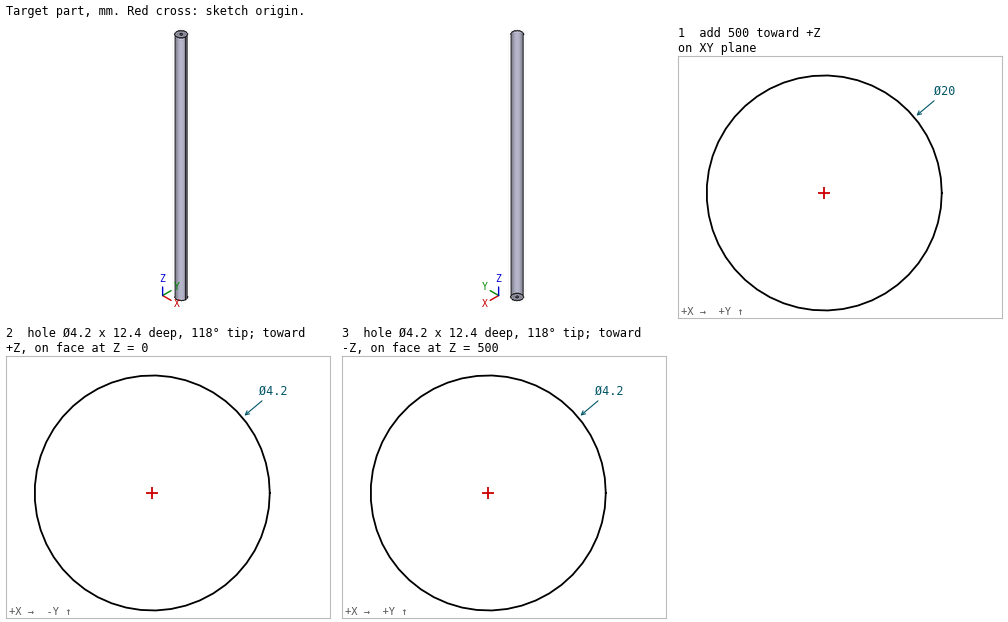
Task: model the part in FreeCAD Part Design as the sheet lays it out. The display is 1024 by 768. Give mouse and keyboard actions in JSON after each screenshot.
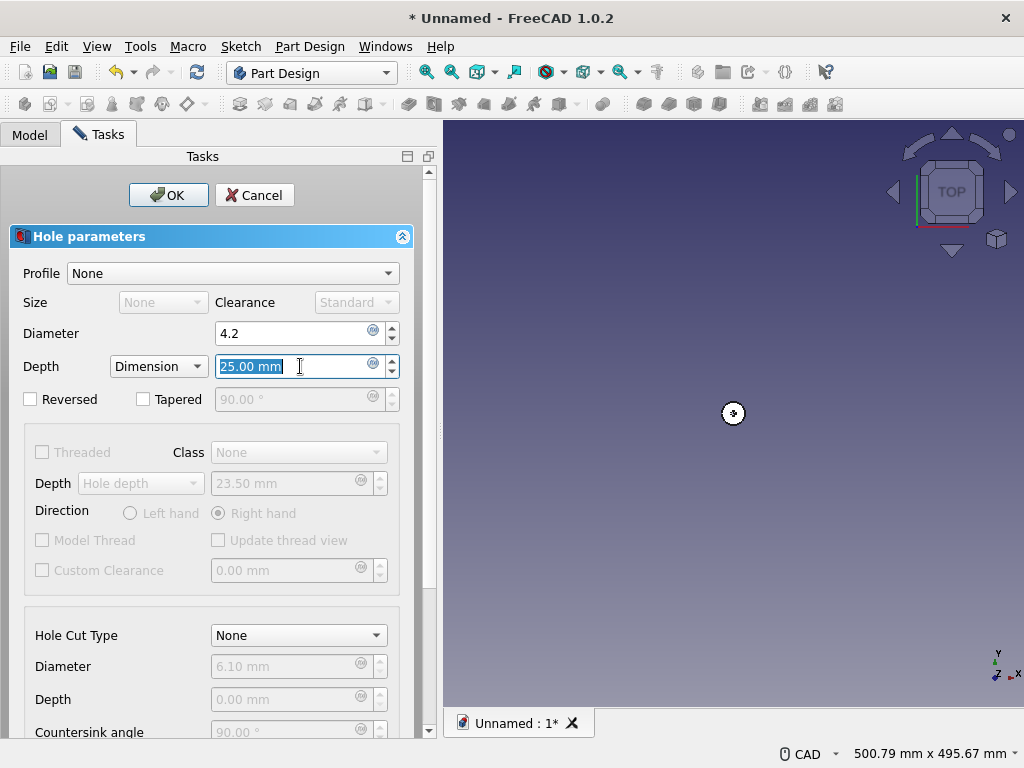
{"action": "type", "text": "12.4"}
{"action": "key", "text": "Tab"}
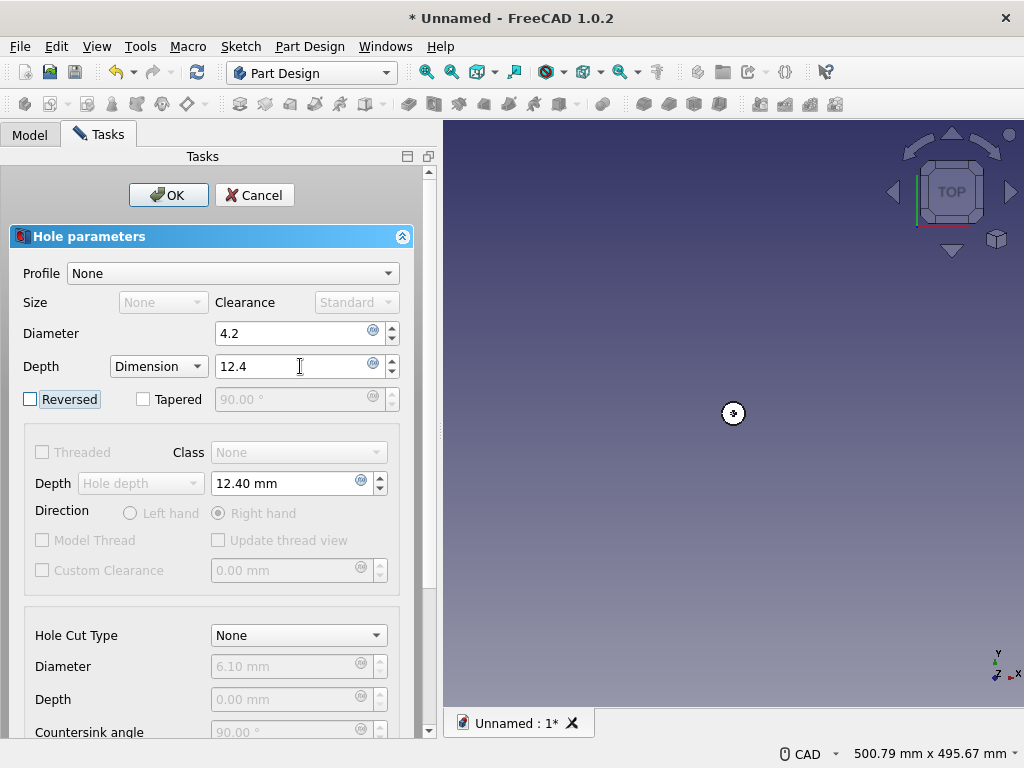
{"action": "left_click", "coordinate": [169, 195]}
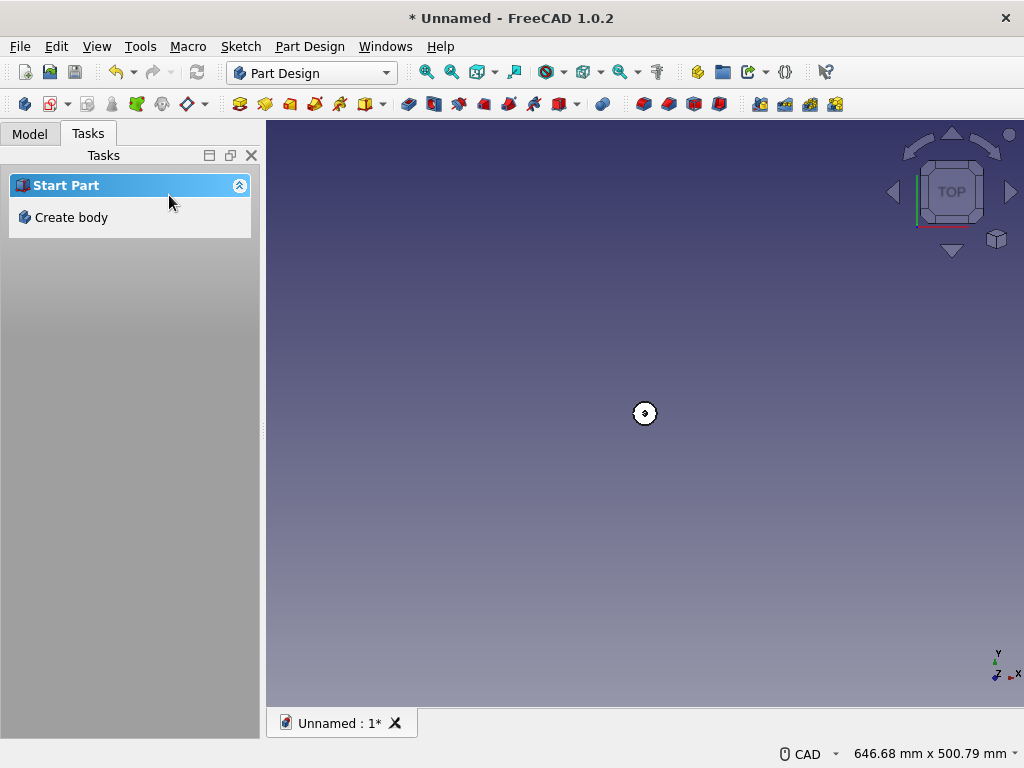
{"action": "key", "text": "0"}